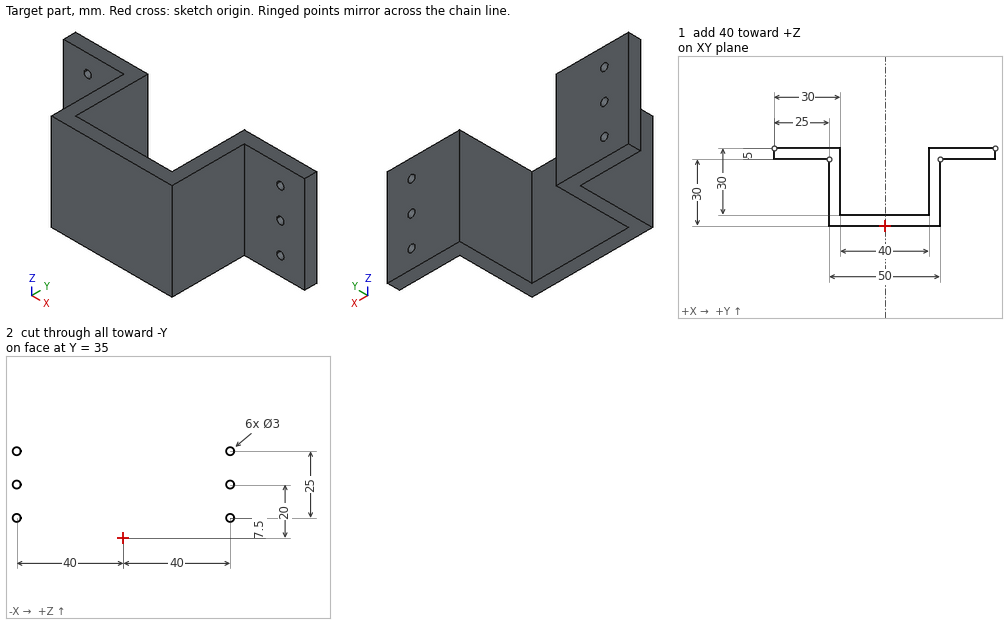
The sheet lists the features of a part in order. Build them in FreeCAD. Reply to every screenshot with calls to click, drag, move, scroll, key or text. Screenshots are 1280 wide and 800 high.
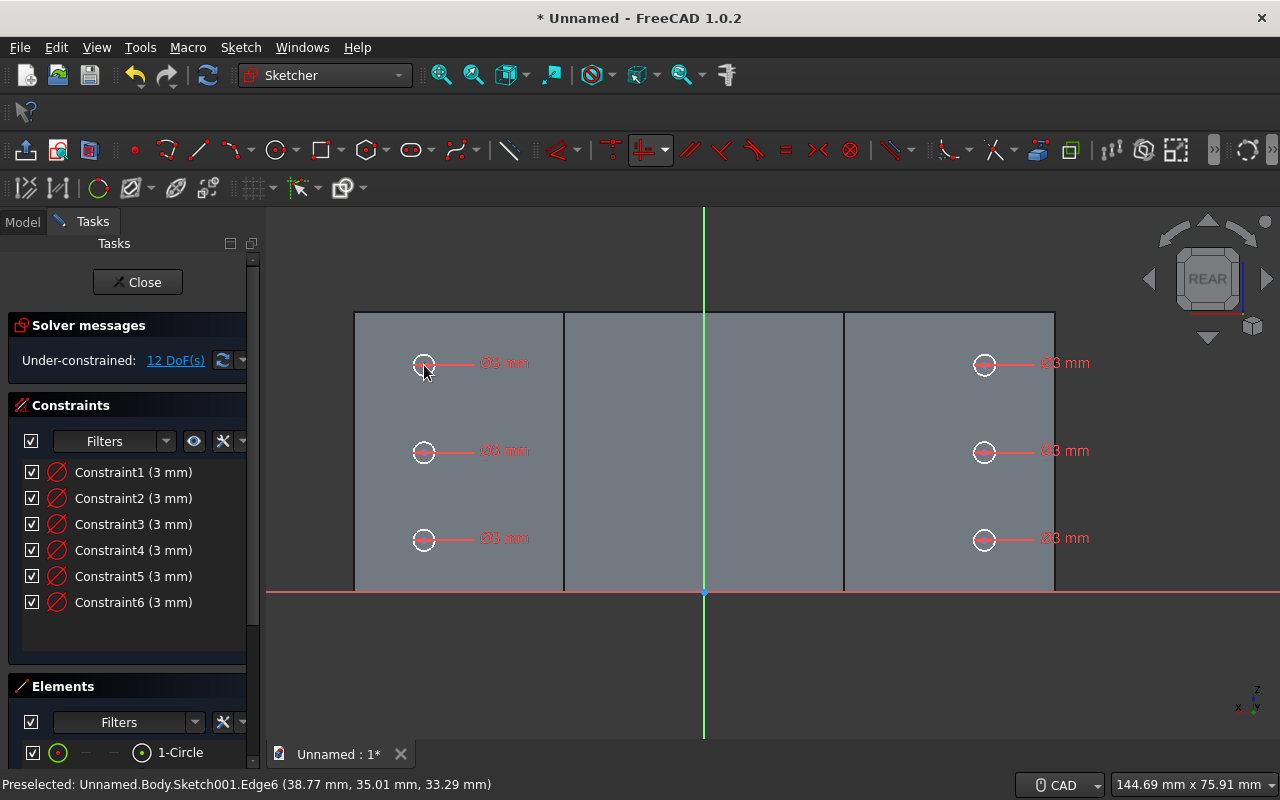
click(984, 540)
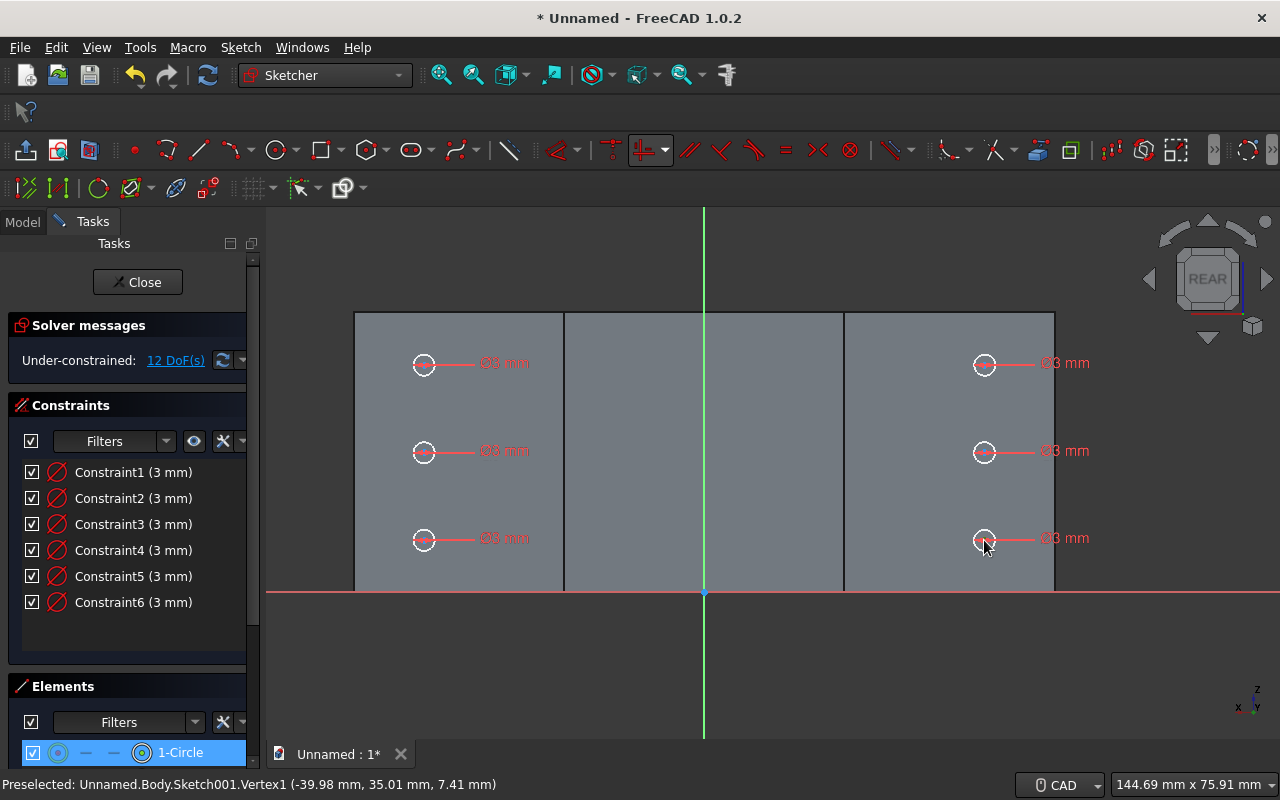
click(984, 453)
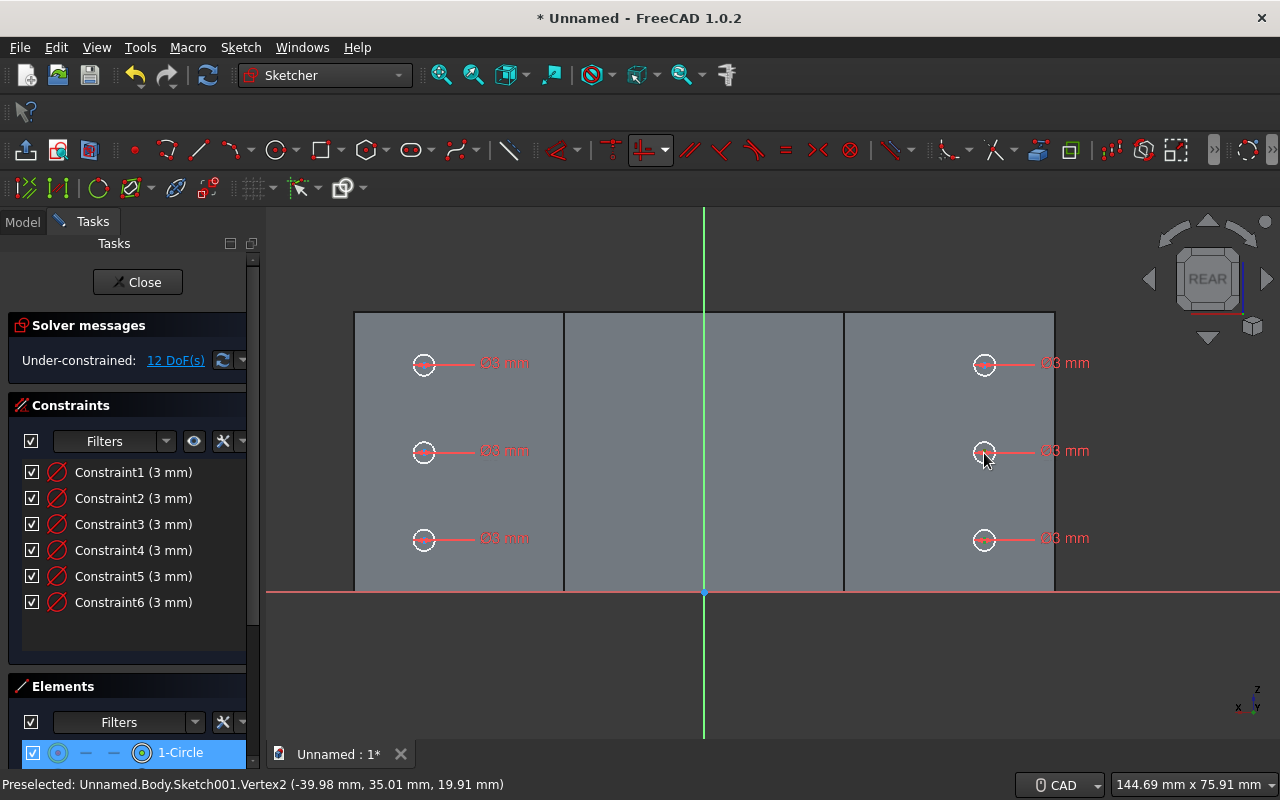
key(v)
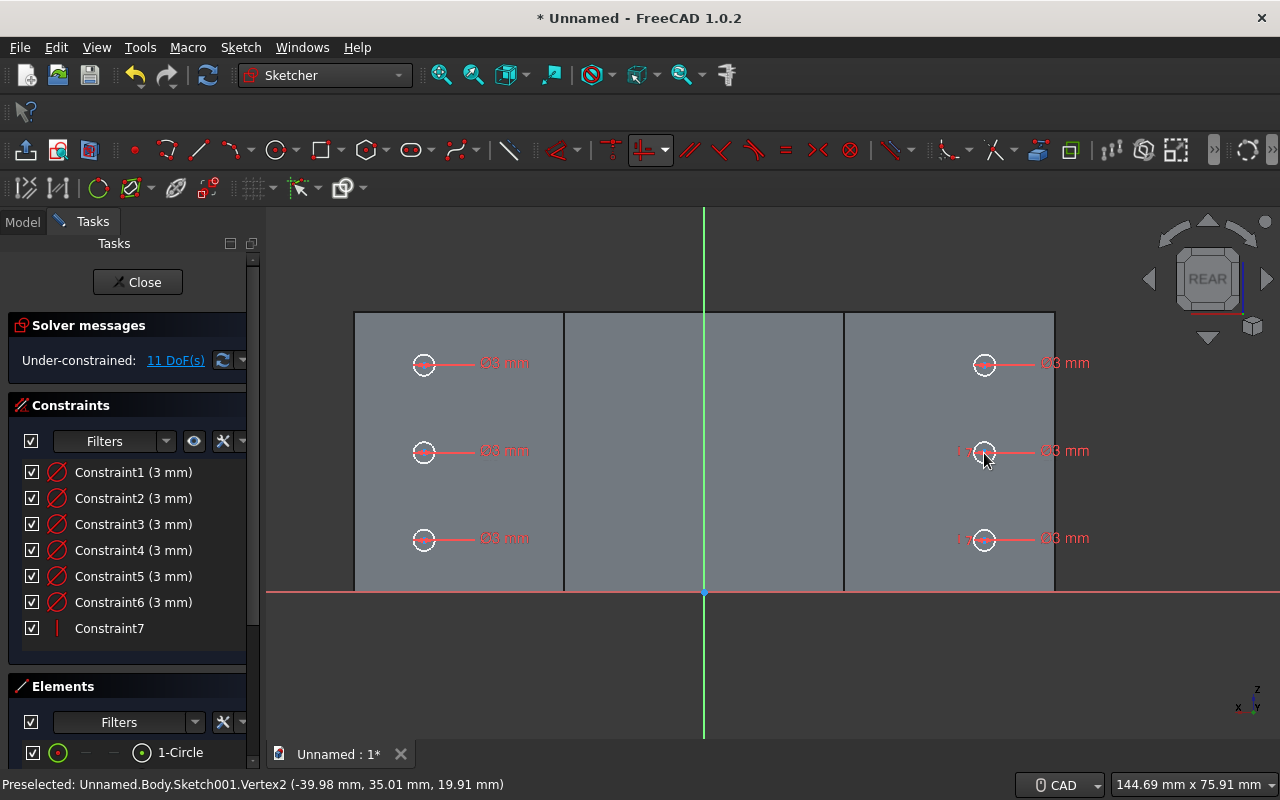
click(984, 453)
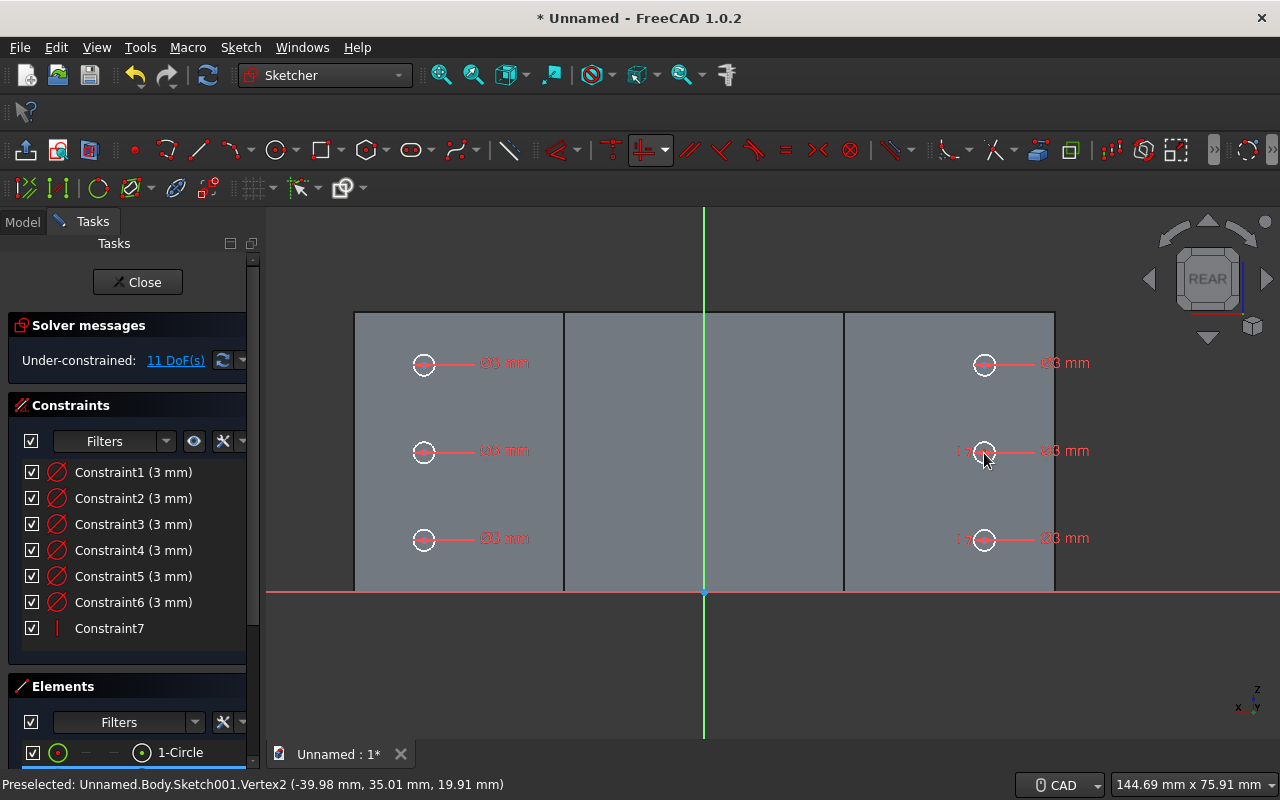
click(985, 365)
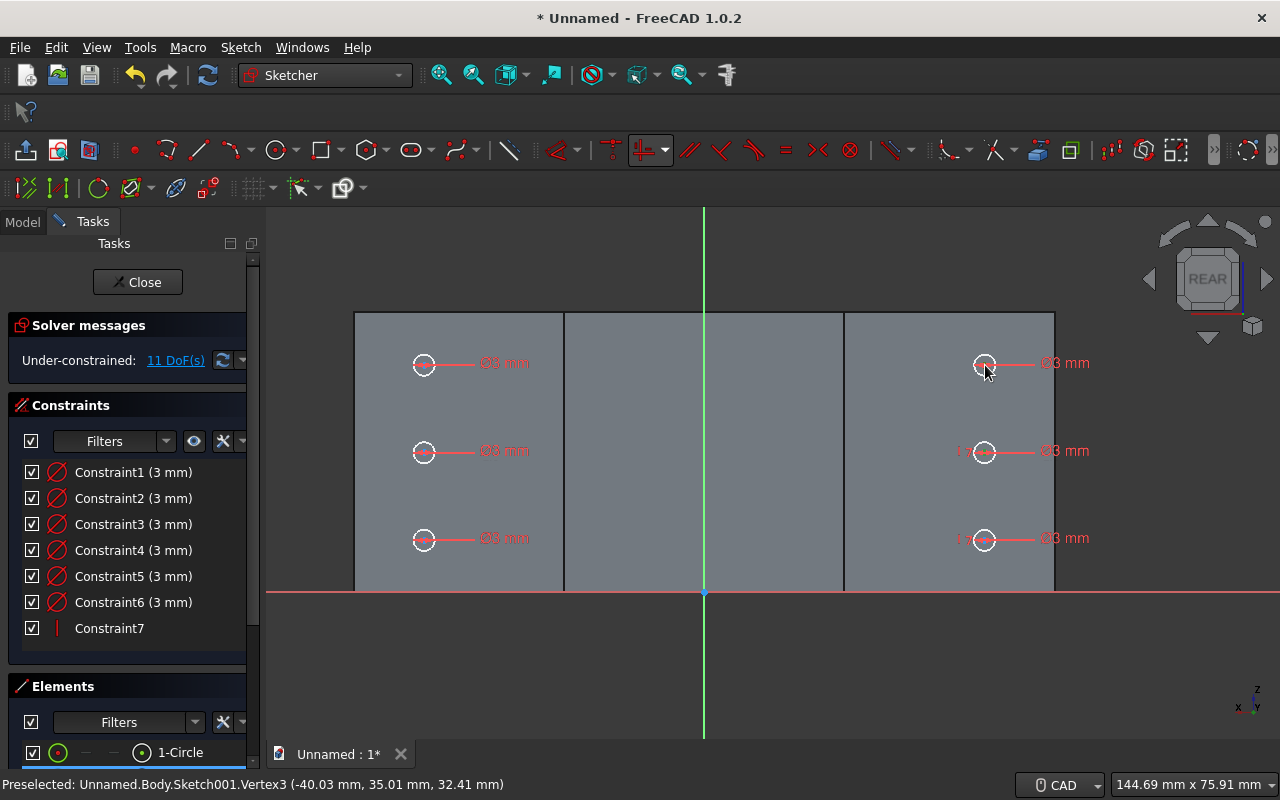
key(v)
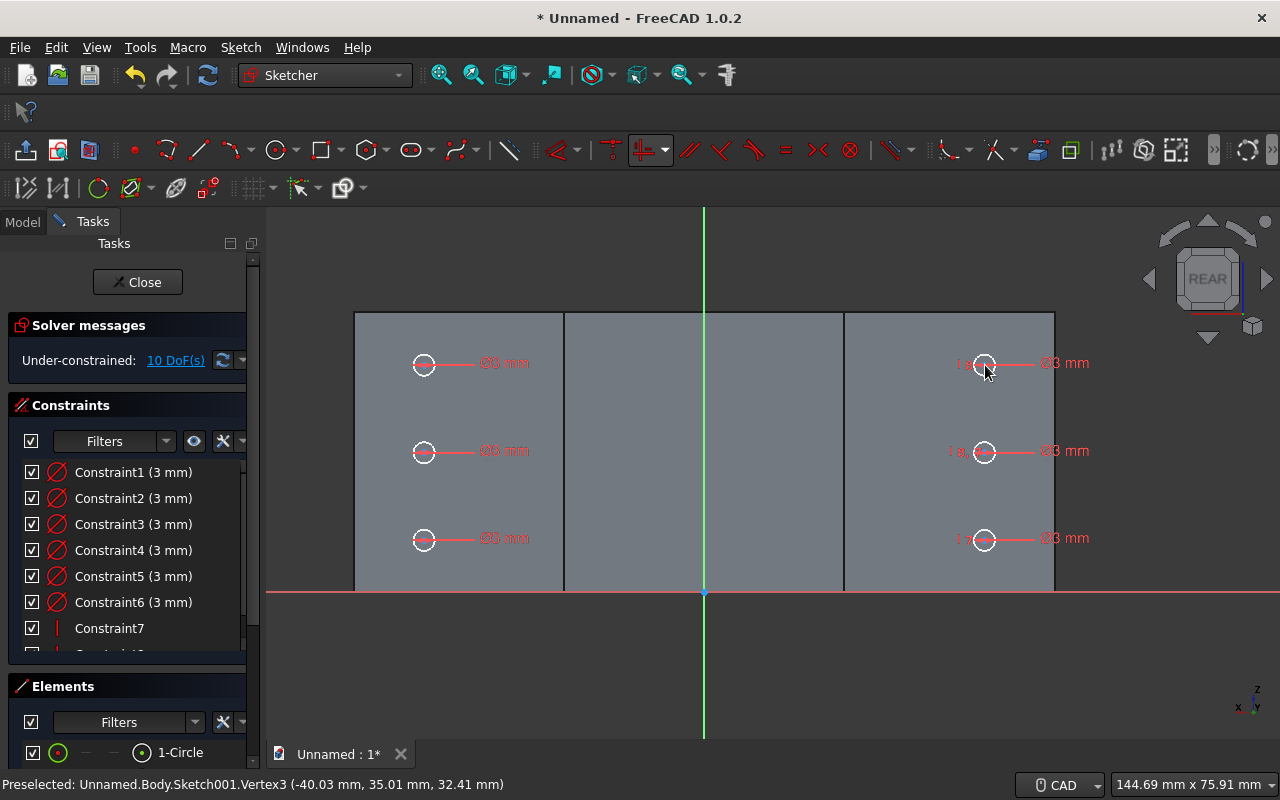
click(984, 540)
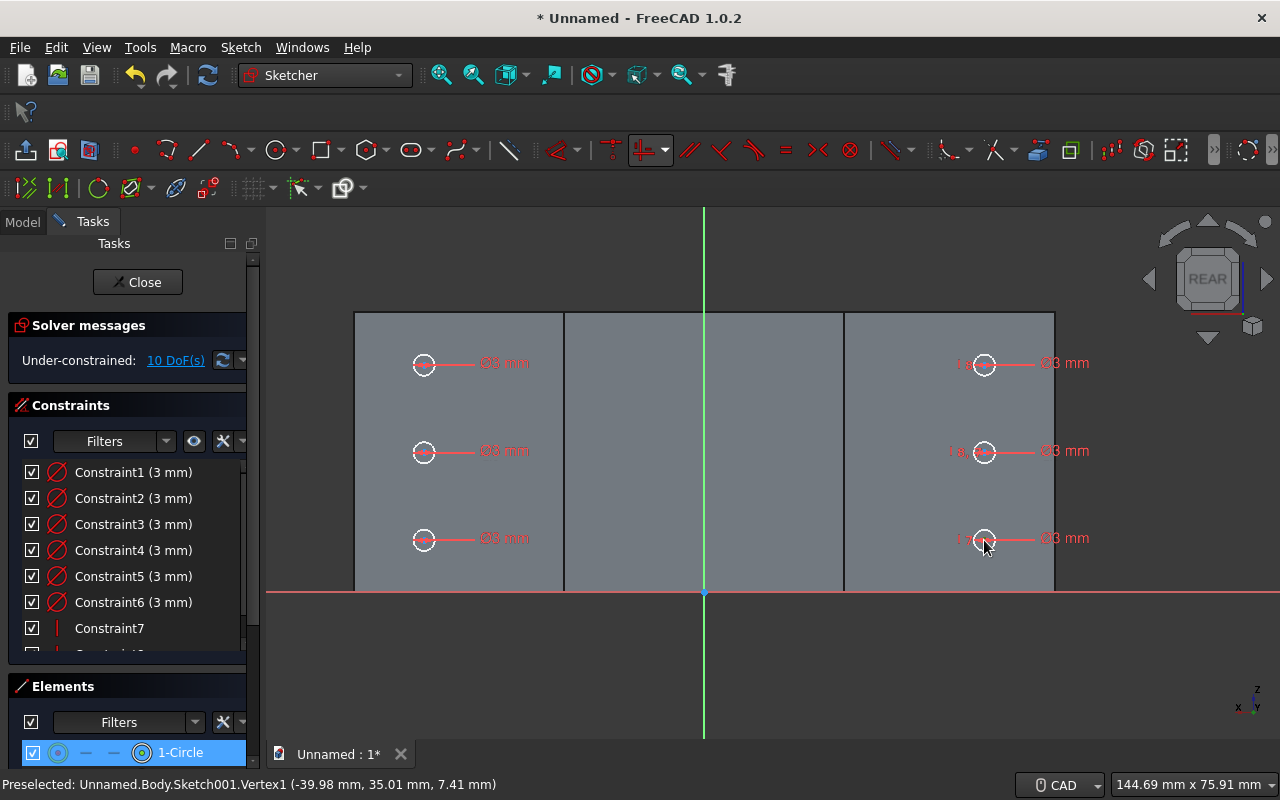
click(424, 540)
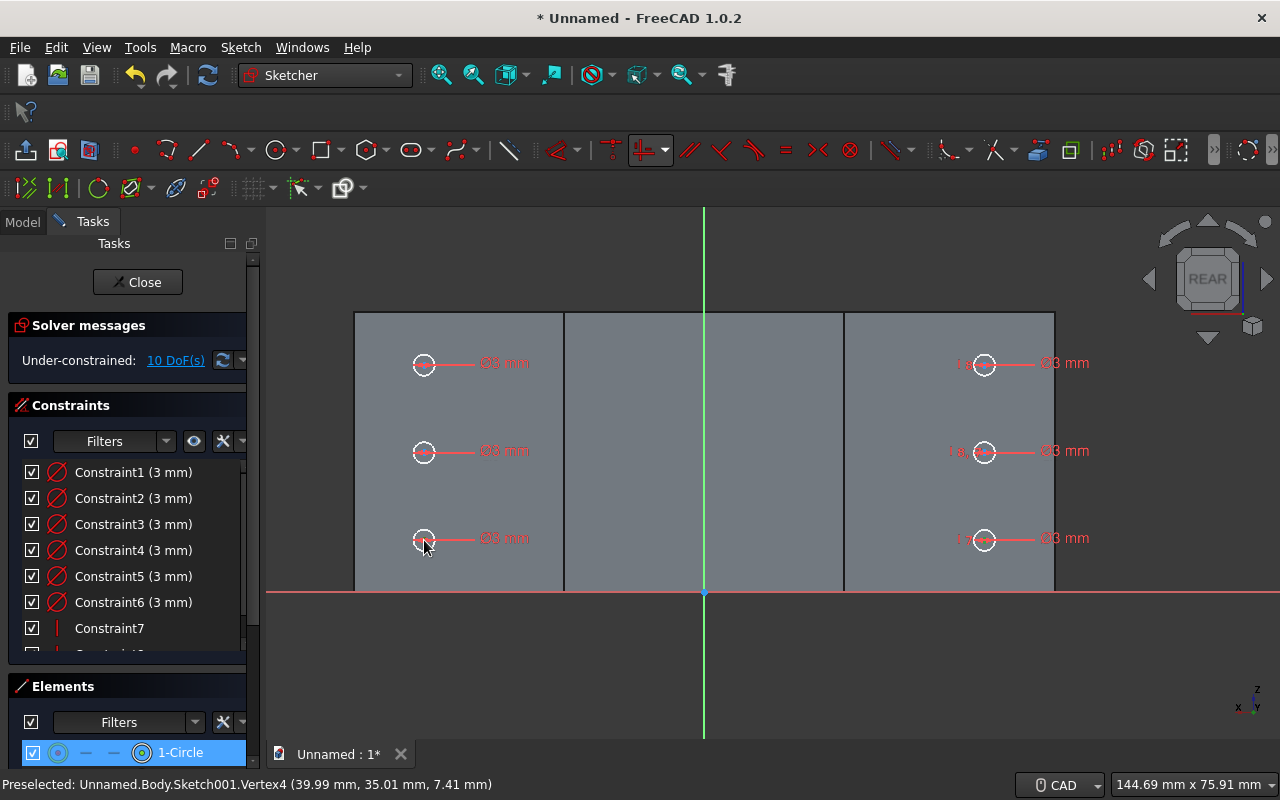
key(h)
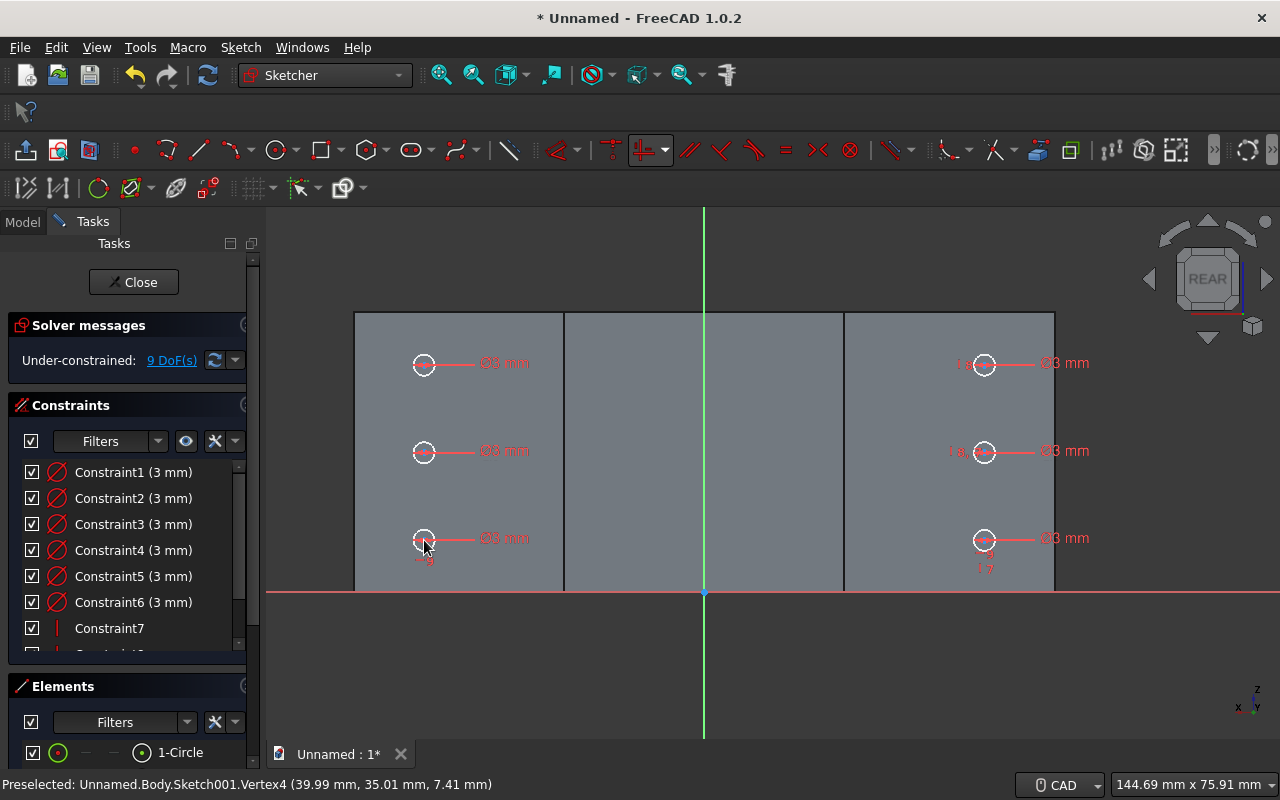
click(424, 540)